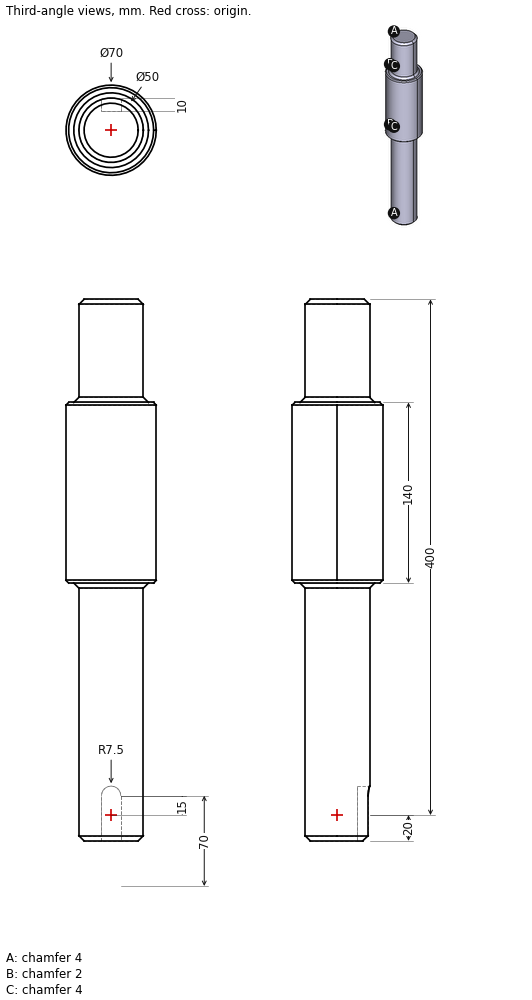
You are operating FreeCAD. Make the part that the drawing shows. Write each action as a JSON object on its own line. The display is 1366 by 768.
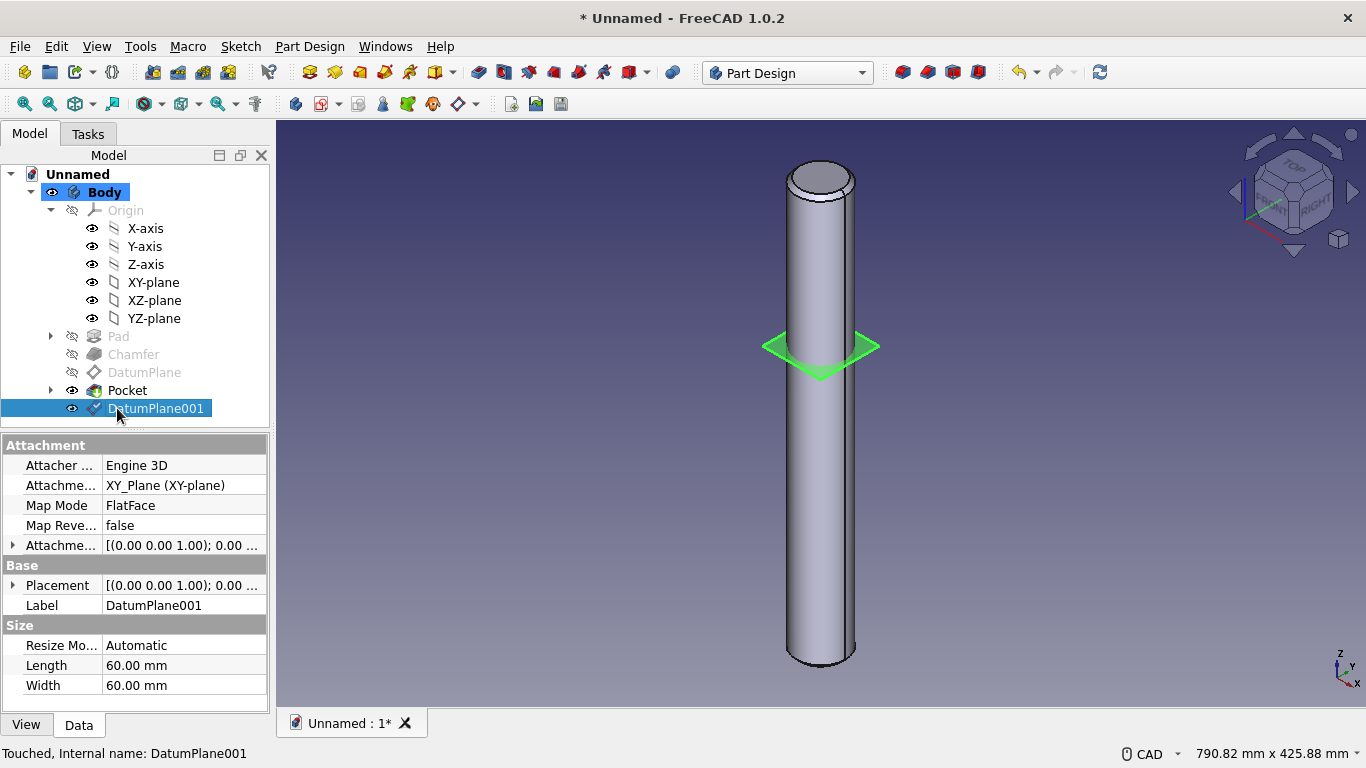
{"action": "left_click", "coordinate": [320, 104]}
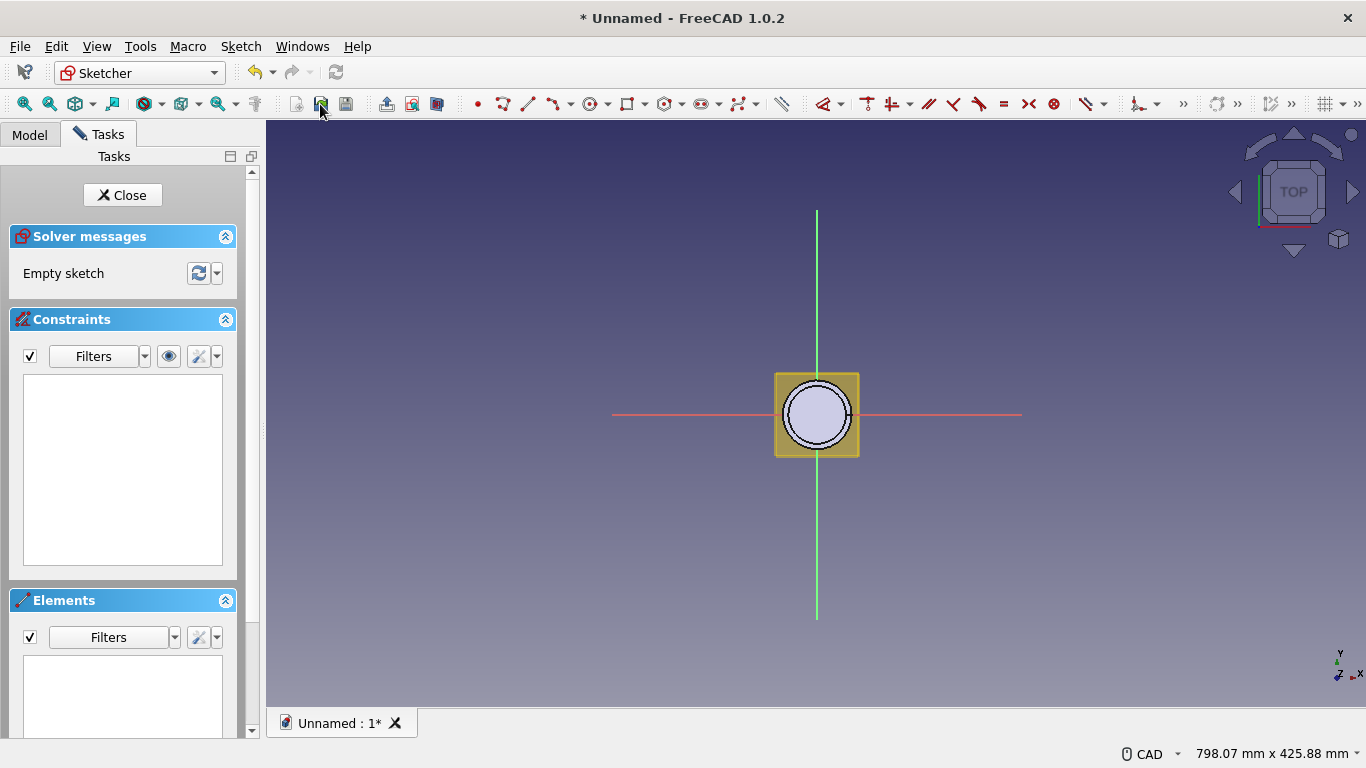
{"action": "left_click", "coordinate": [437, 104]}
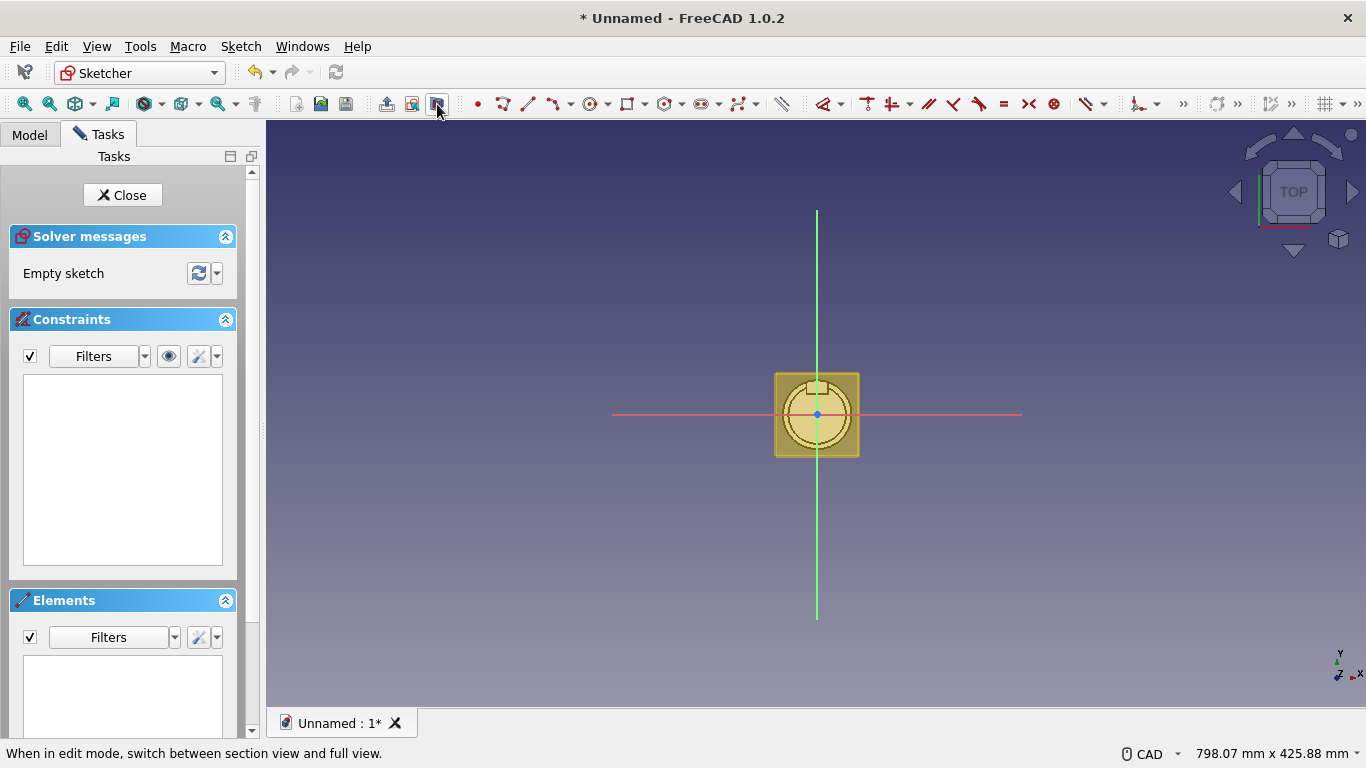
{"action": "scroll", "coordinate": [840, 415], "scroll_direction": "up", "scroll_amount": 7}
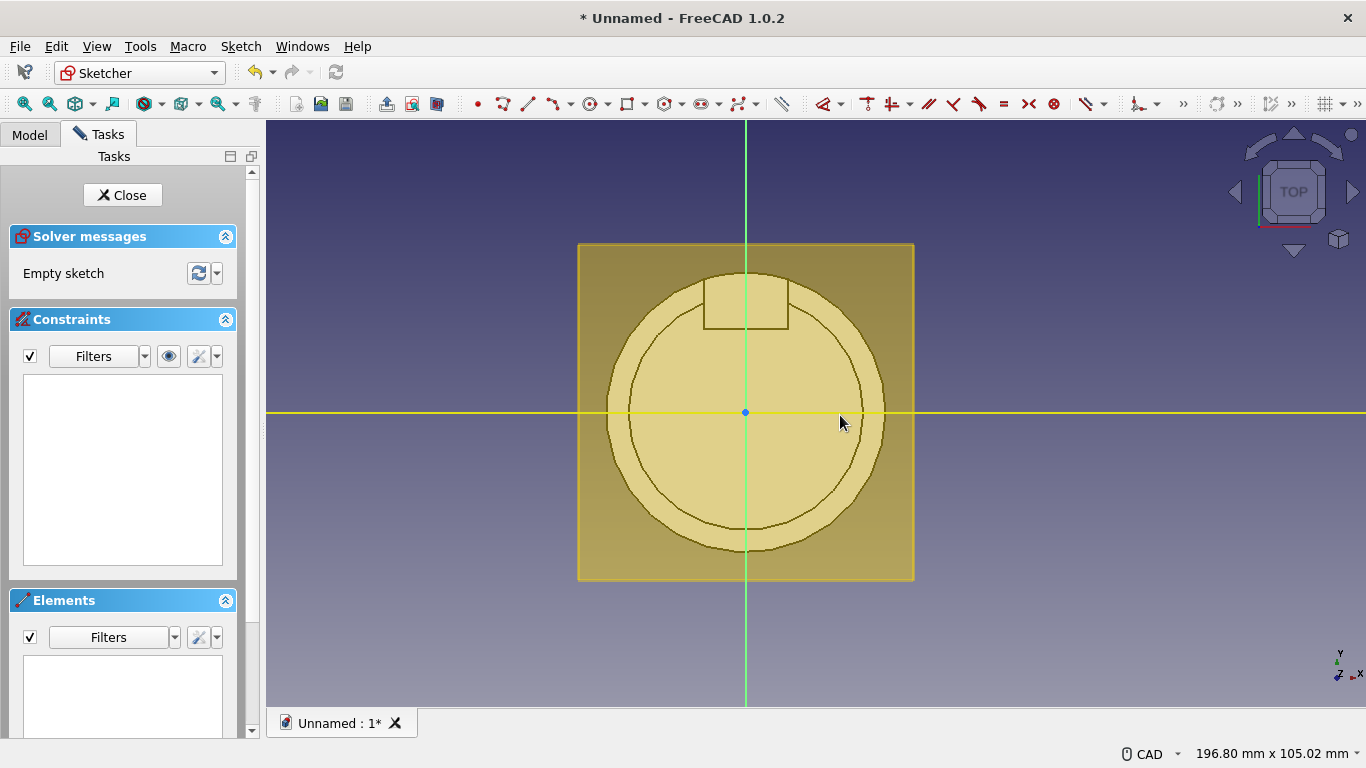
{"action": "left_click", "coordinate": [590, 104]}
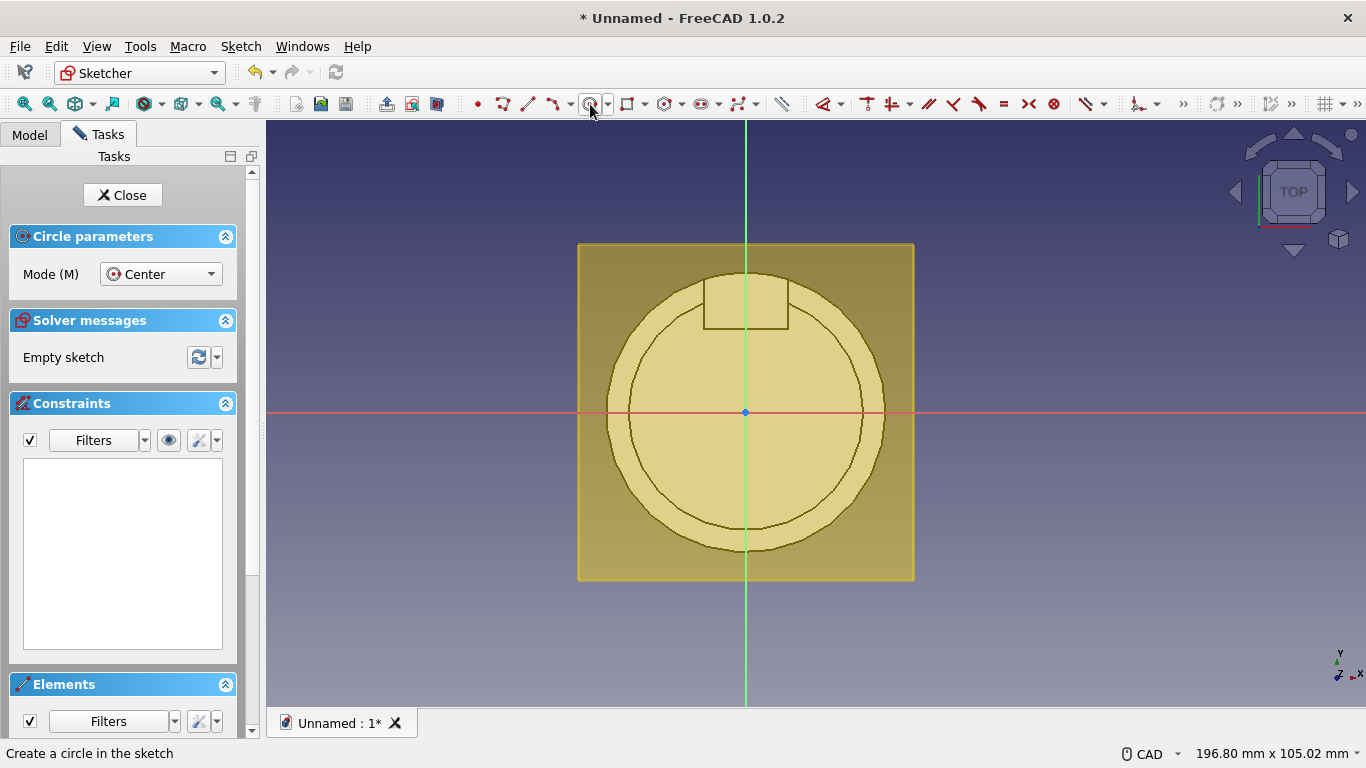
{"action": "left_click", "coordinate": [746, 413]}
{"action": "left_click", "coordinate": [884, 274]}
{"action": "key", "text": "Escape"}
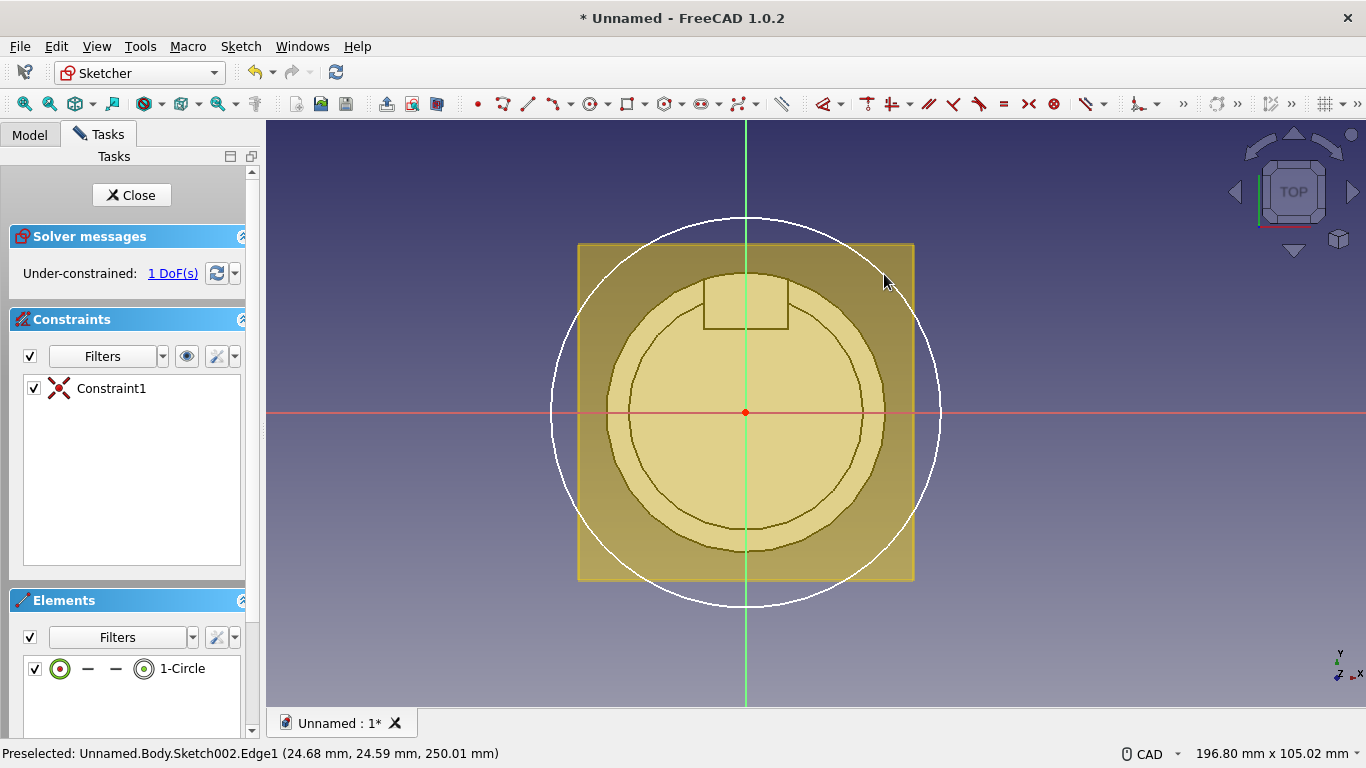
{"action": "left_click", "coordinate": [822, 104]}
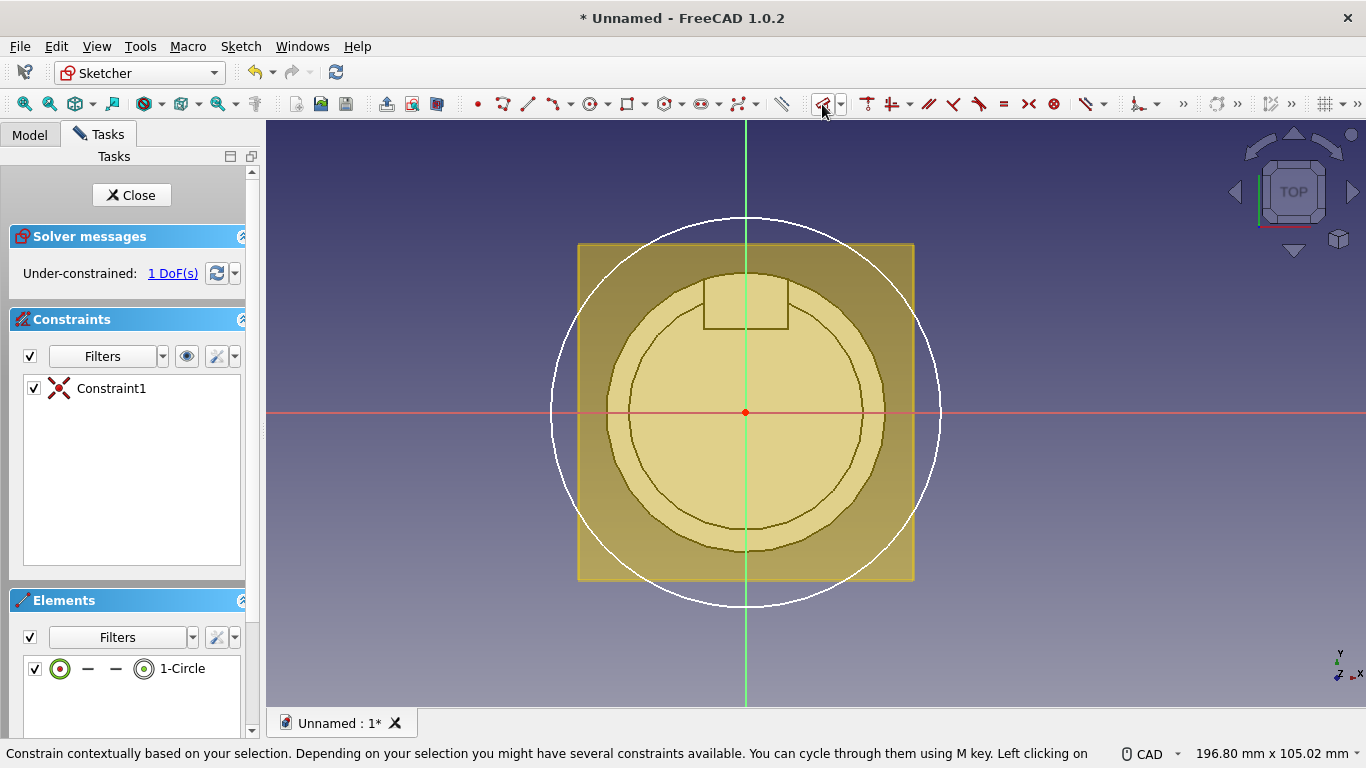
{"action": "left_click", "coordinate": [883, 274]}
{"action": "left_click", "coordinate": [906, 251]}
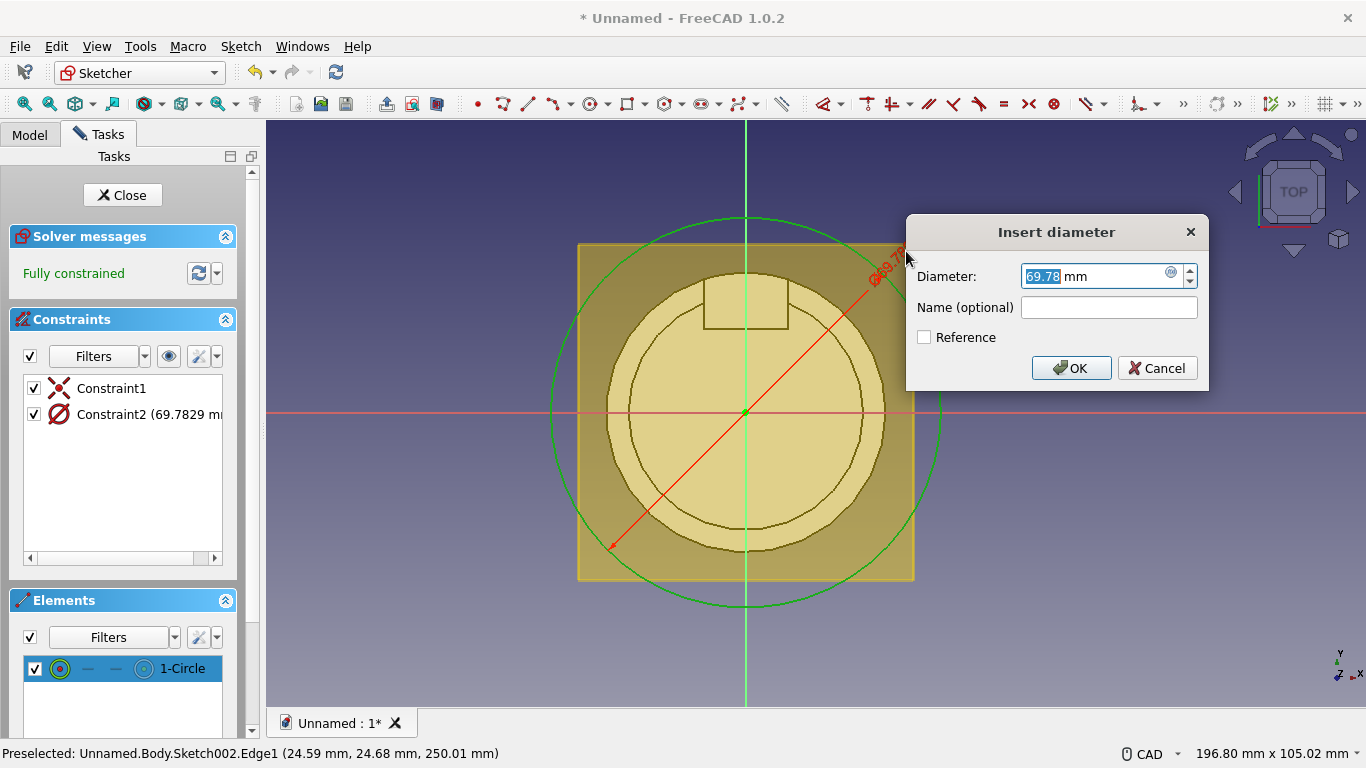
{"action": "type", "text": "70"}
{"action": "key", "text": "Return"}
{"action": "key", "text": "Escape"}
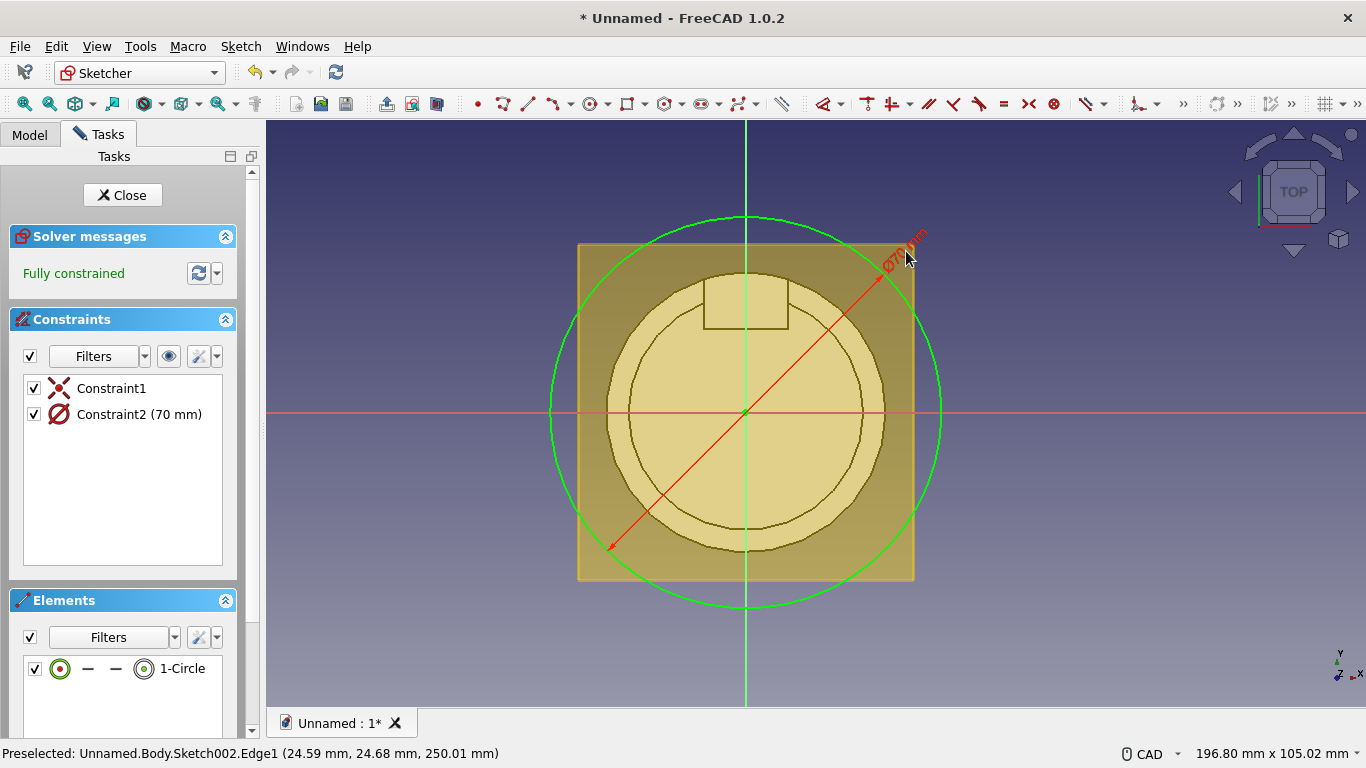
{"action": "left_click", "coordinate": [123, 195]}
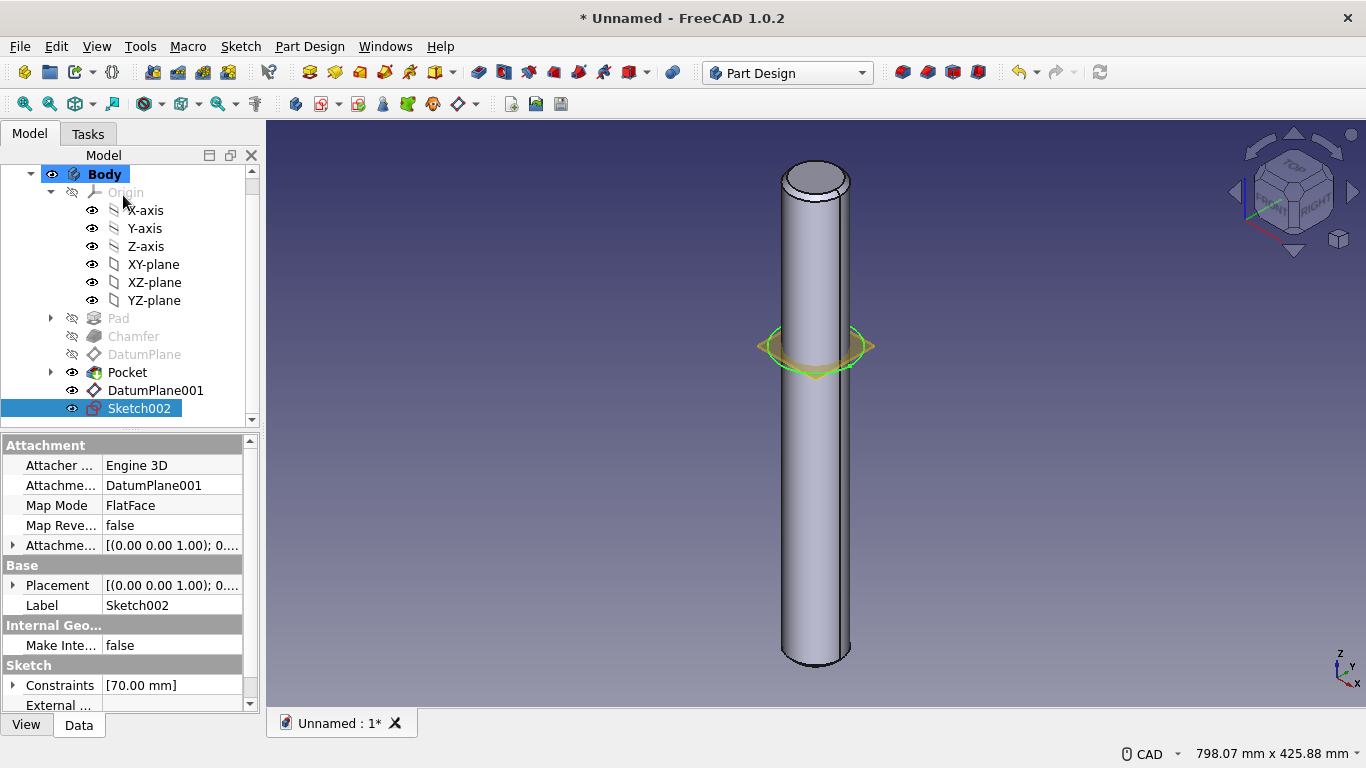
{"action": "left_click", "coordinate": [310, 72]}